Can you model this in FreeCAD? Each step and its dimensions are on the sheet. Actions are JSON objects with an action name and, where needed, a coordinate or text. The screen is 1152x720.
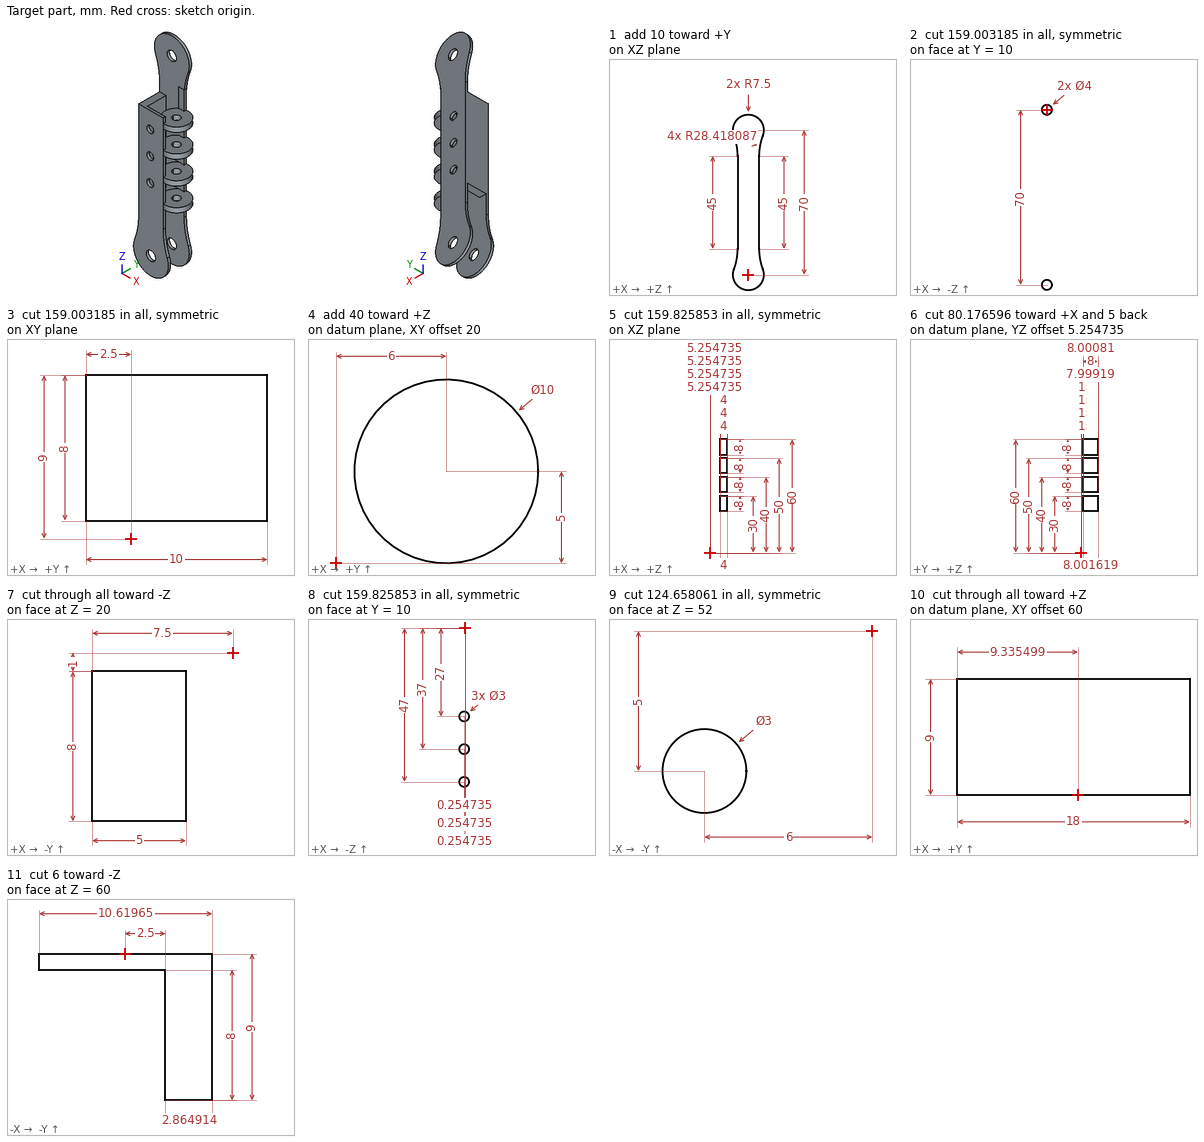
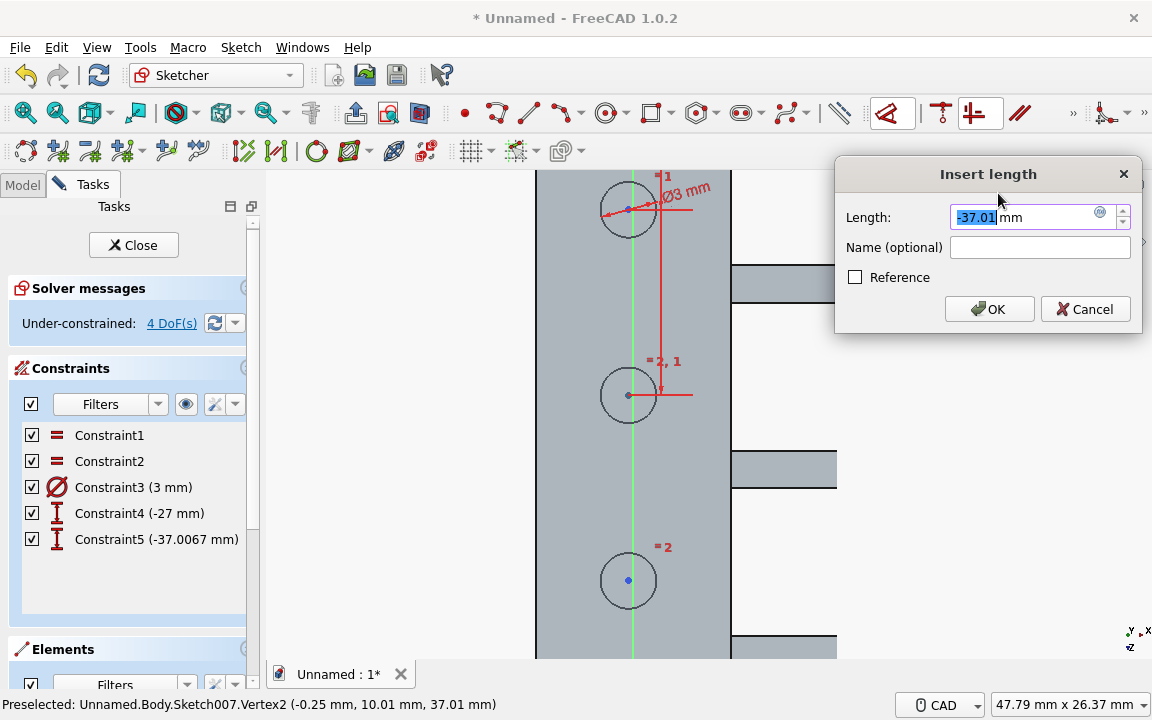
{"action": "type", "text": "-37"}
{"action": "key", "text": "Return"}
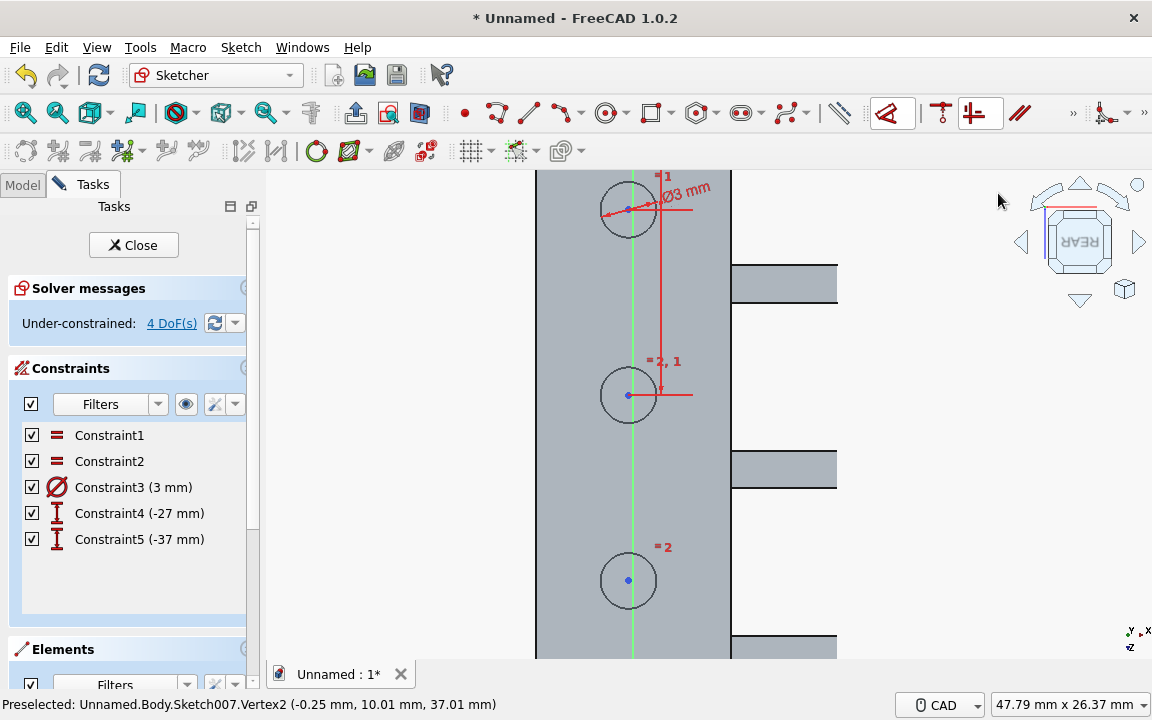
{"action": "left_click", "coordinate": [629, 581]}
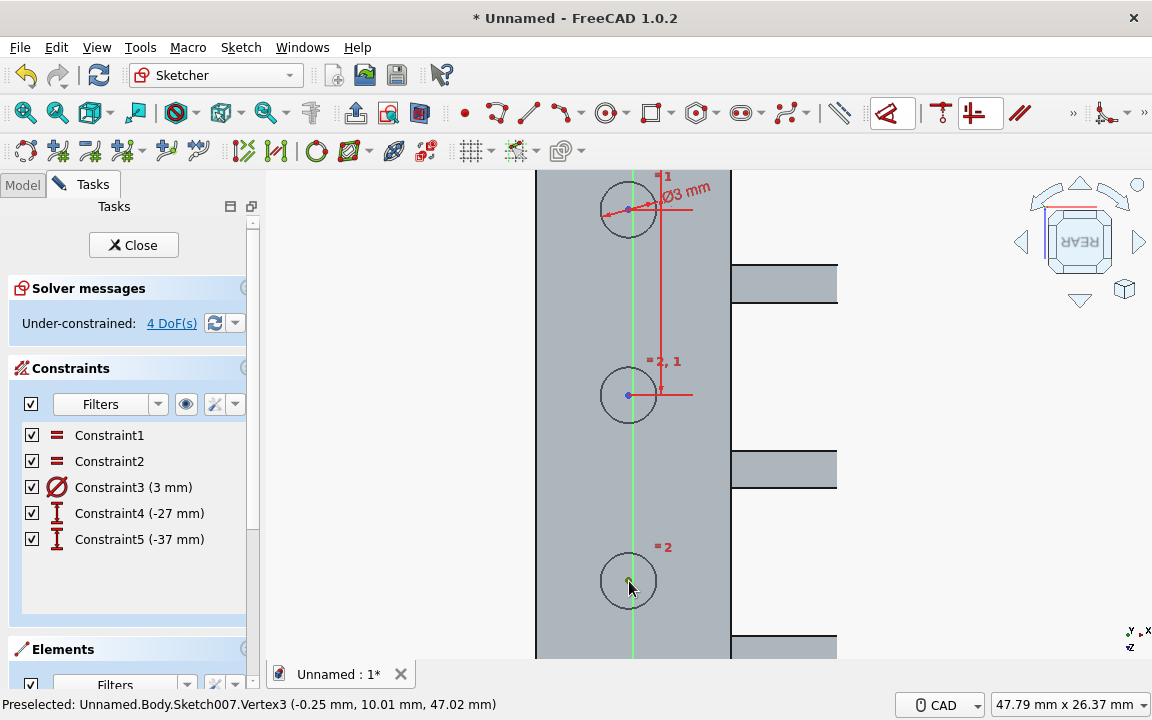
{"action": "left_click", "coordinate": [910, 114]}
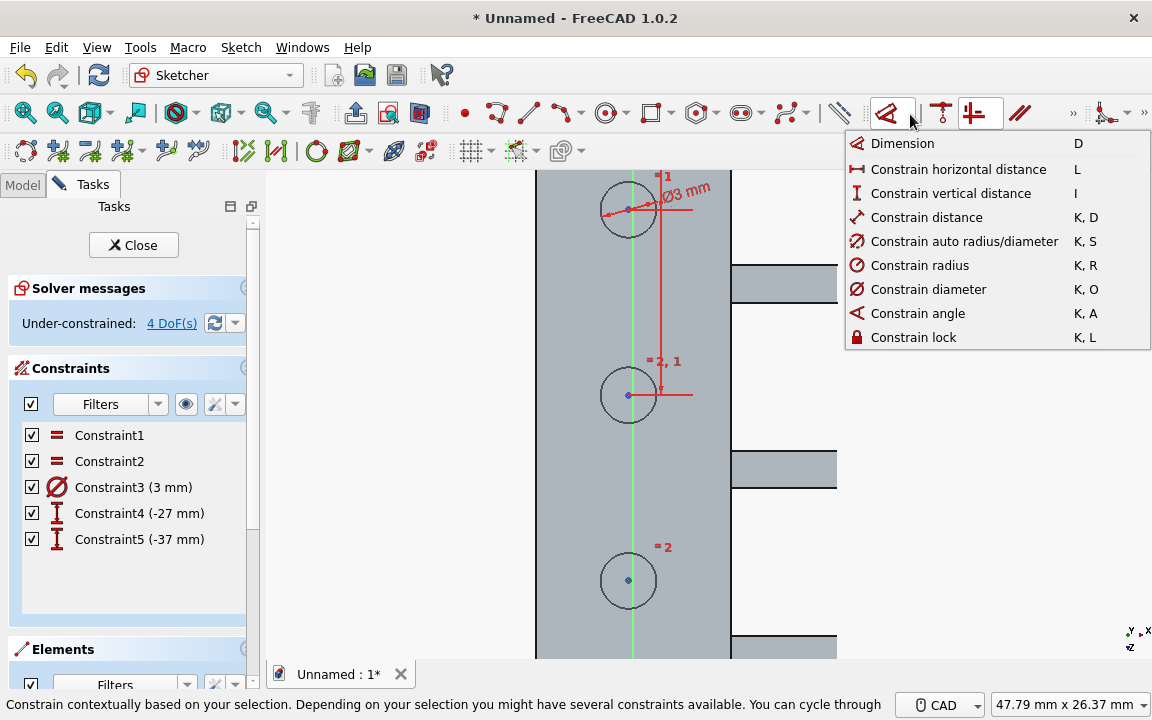
{"action": "left_click", "coordinate": [998, 193]}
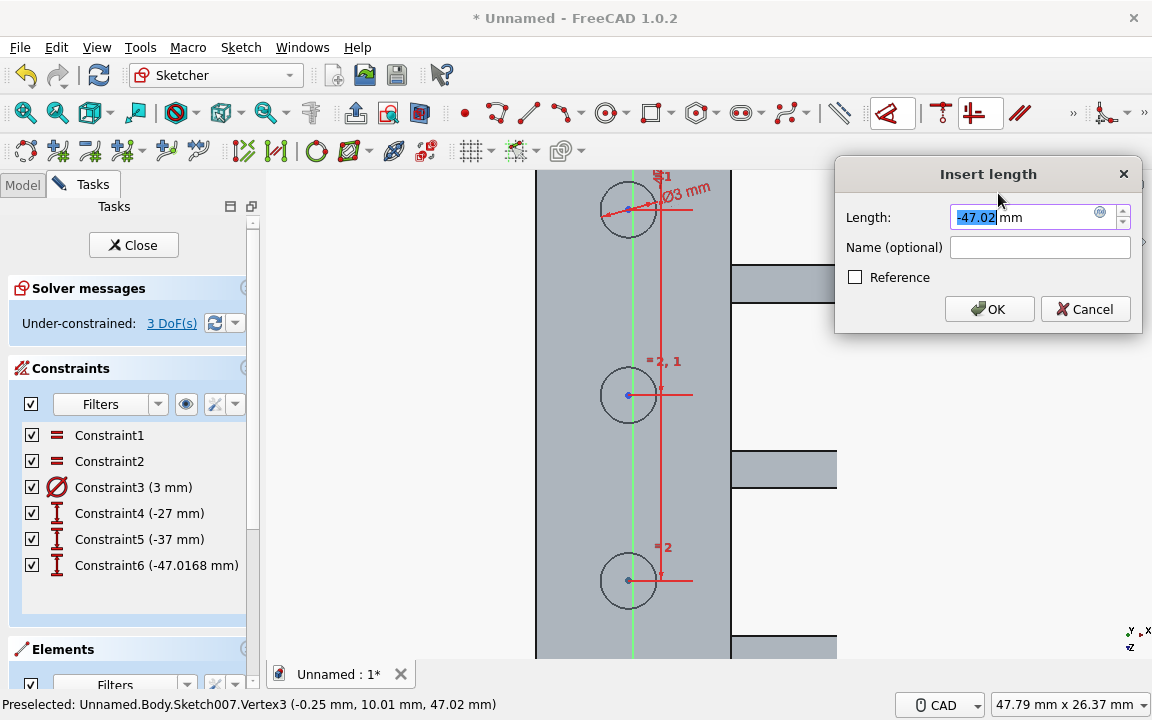
{"action": "type", "text": "-47"}
{"action": "key", "text": "Return"}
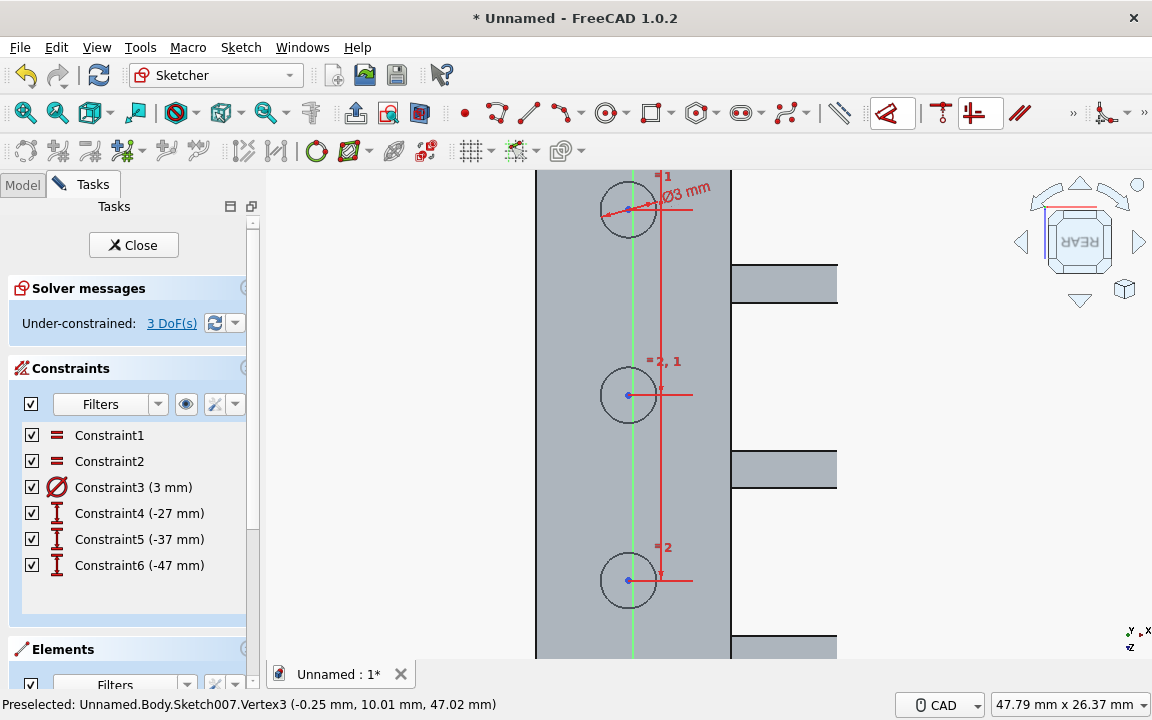
{"action": "scroll", "coordinate": [628, 210], "scroll_direction": "up", "scroll_amount": 11}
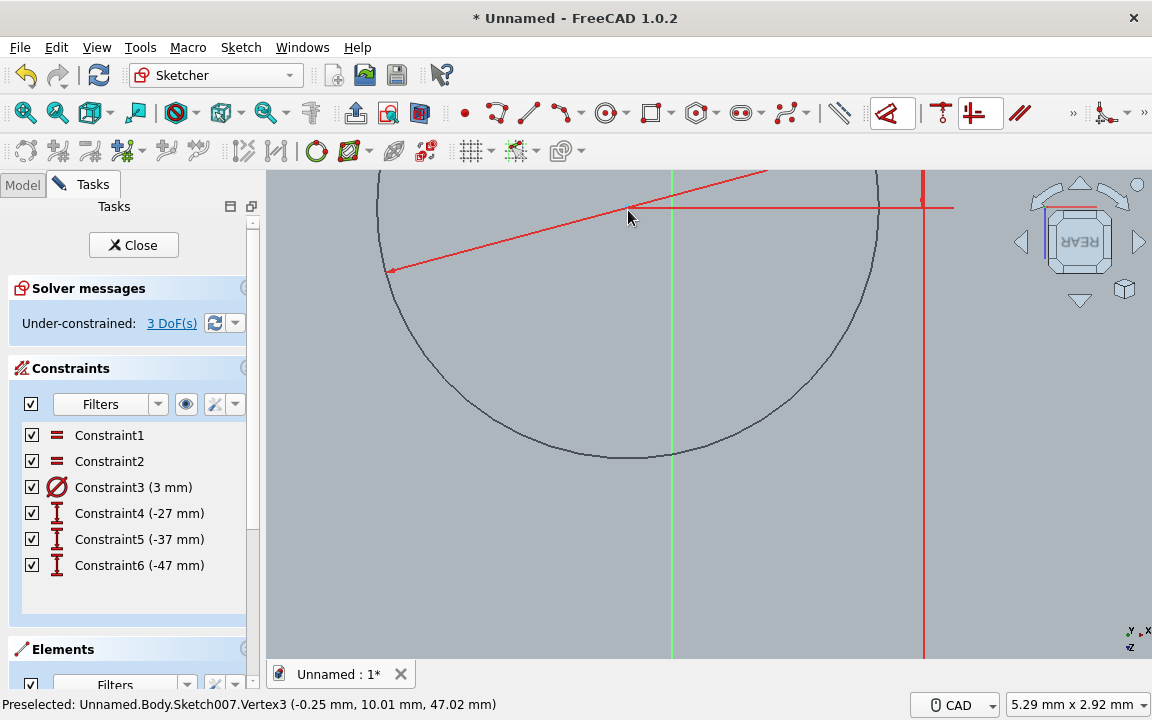
{"action": "left_click", "coordinate": [628, 208]}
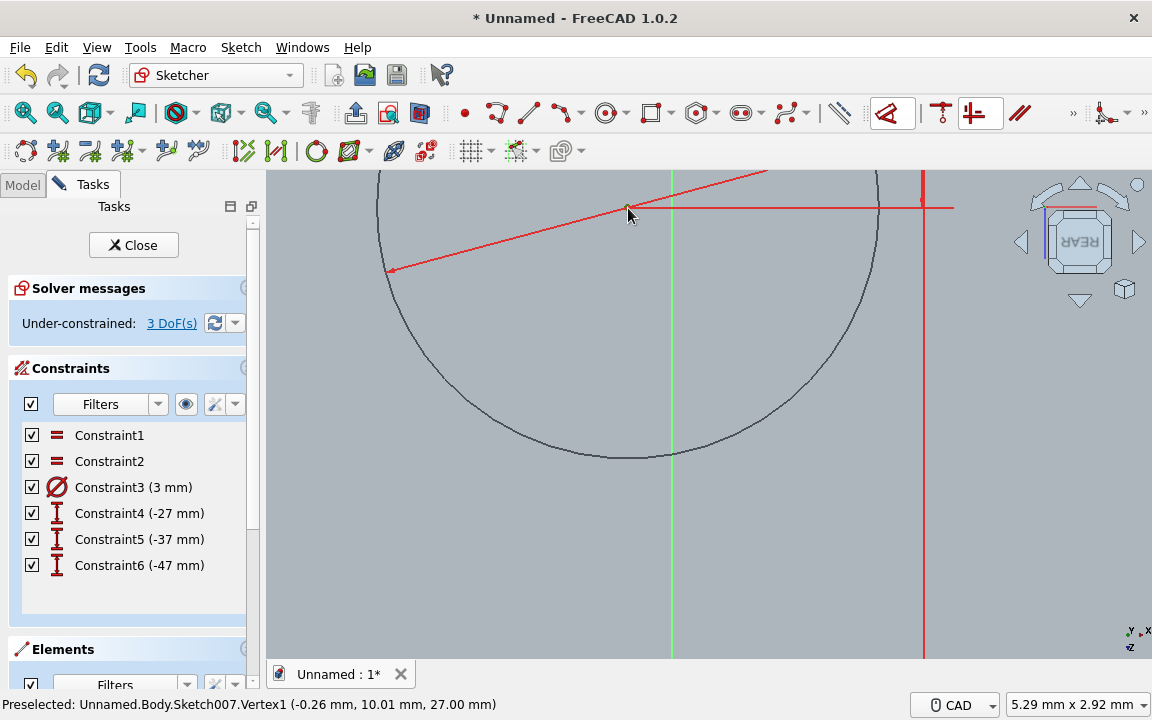
{"action": "key", "text": "l"}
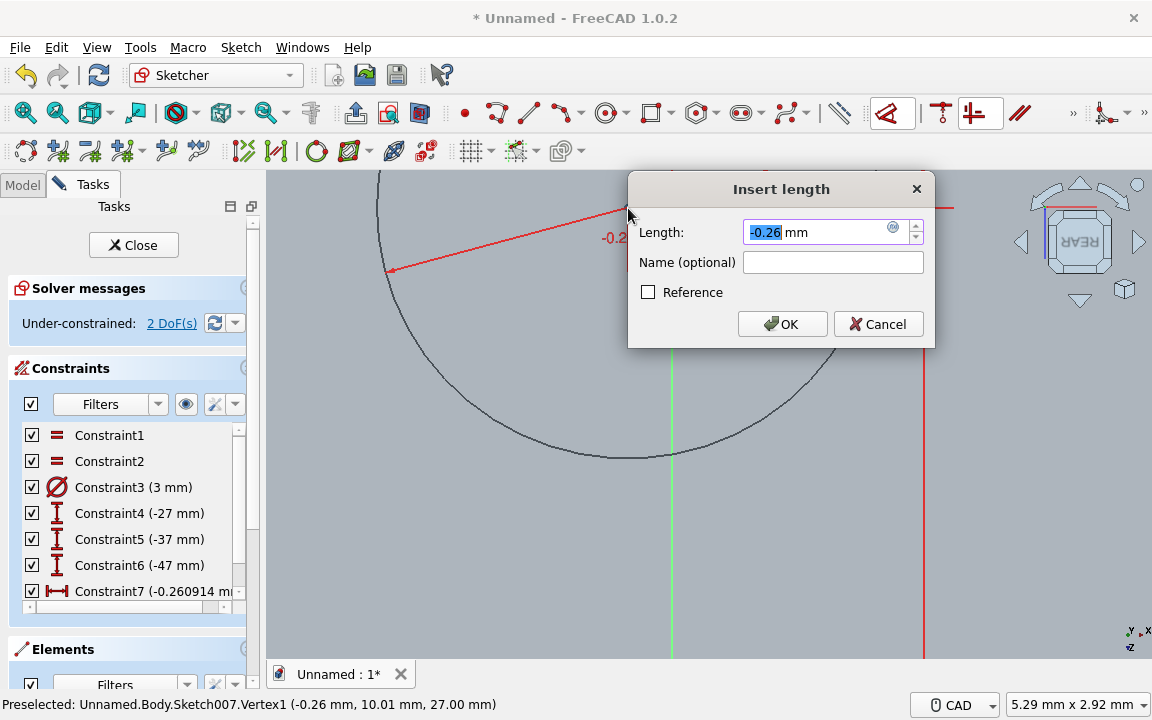
{"action": "type", "text": "-0.254735"}
{"action": "key", "text": "Return"}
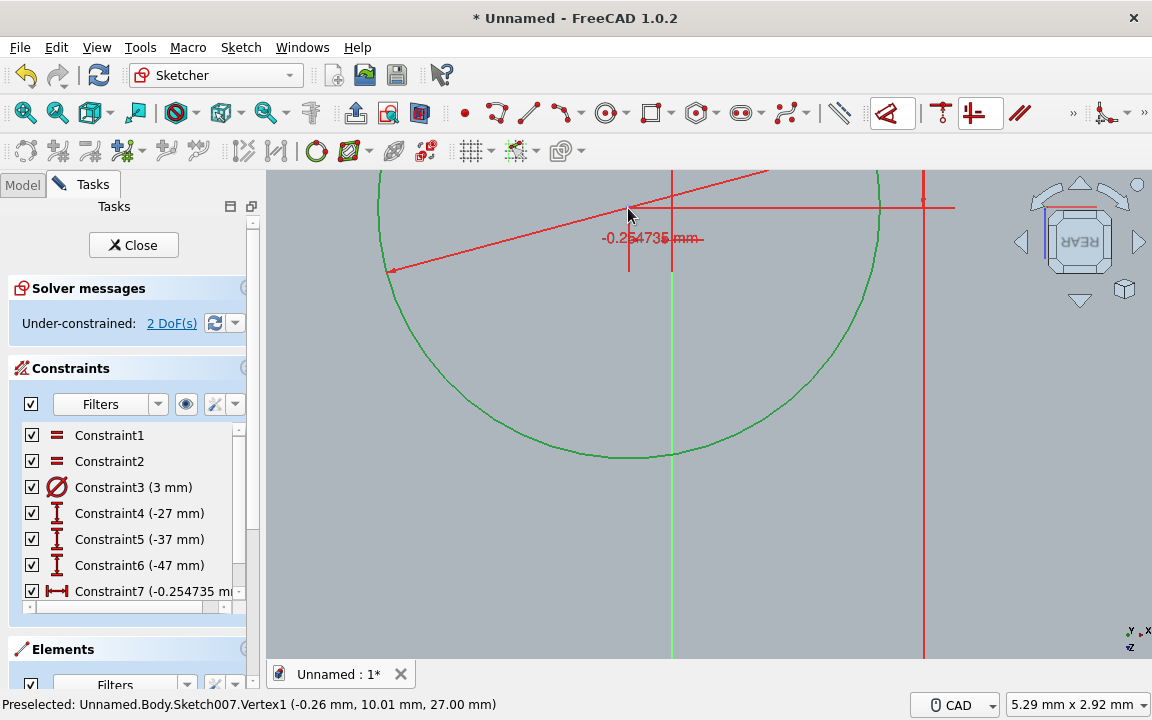
{"action": "scroll", "coordinate": [641, 443], "scroll_direction": "down", "scroll_amount": 16}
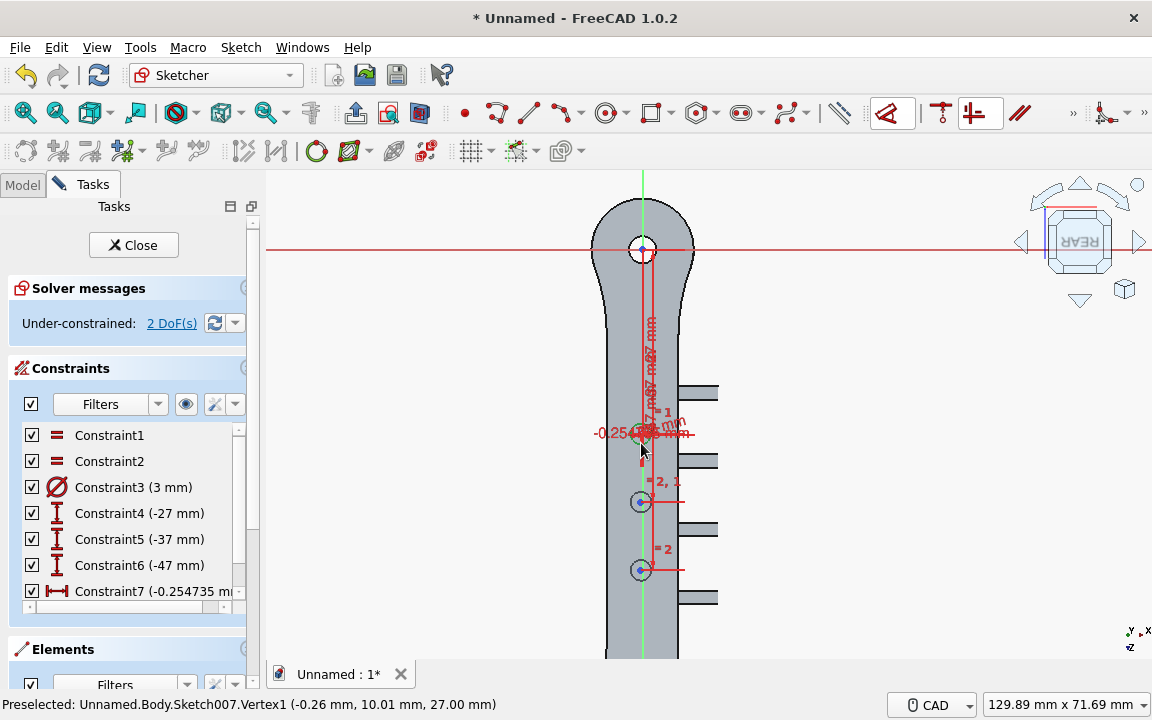
{"action": "scroll", "coordinate": [641, 502], "scroll_direction": "up", "scroll_amount": 16}